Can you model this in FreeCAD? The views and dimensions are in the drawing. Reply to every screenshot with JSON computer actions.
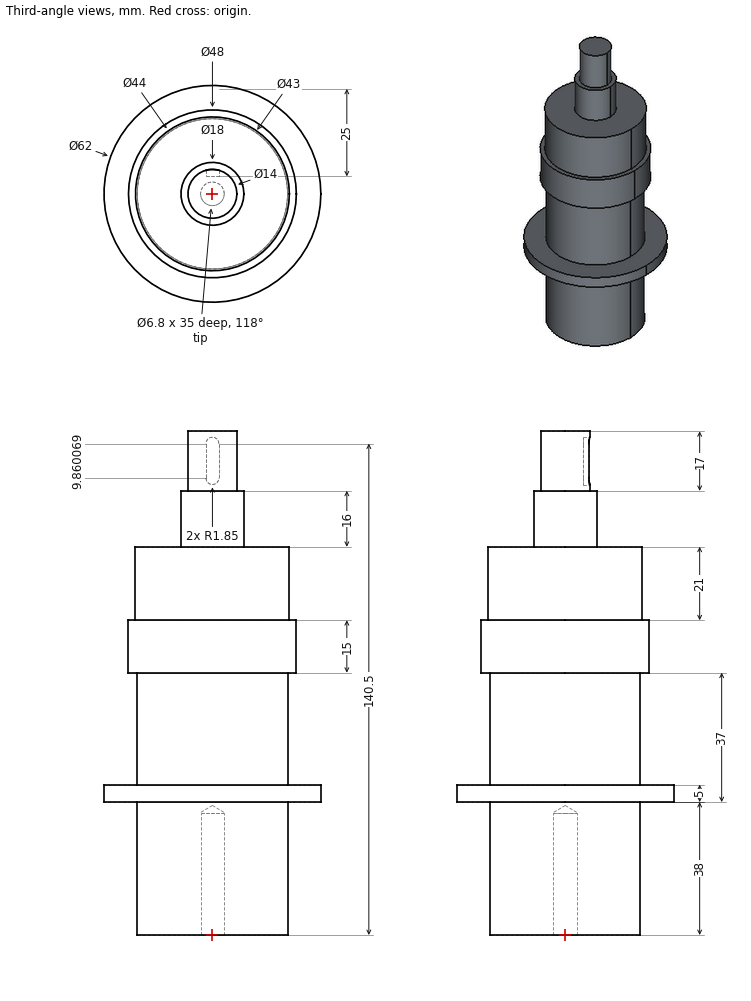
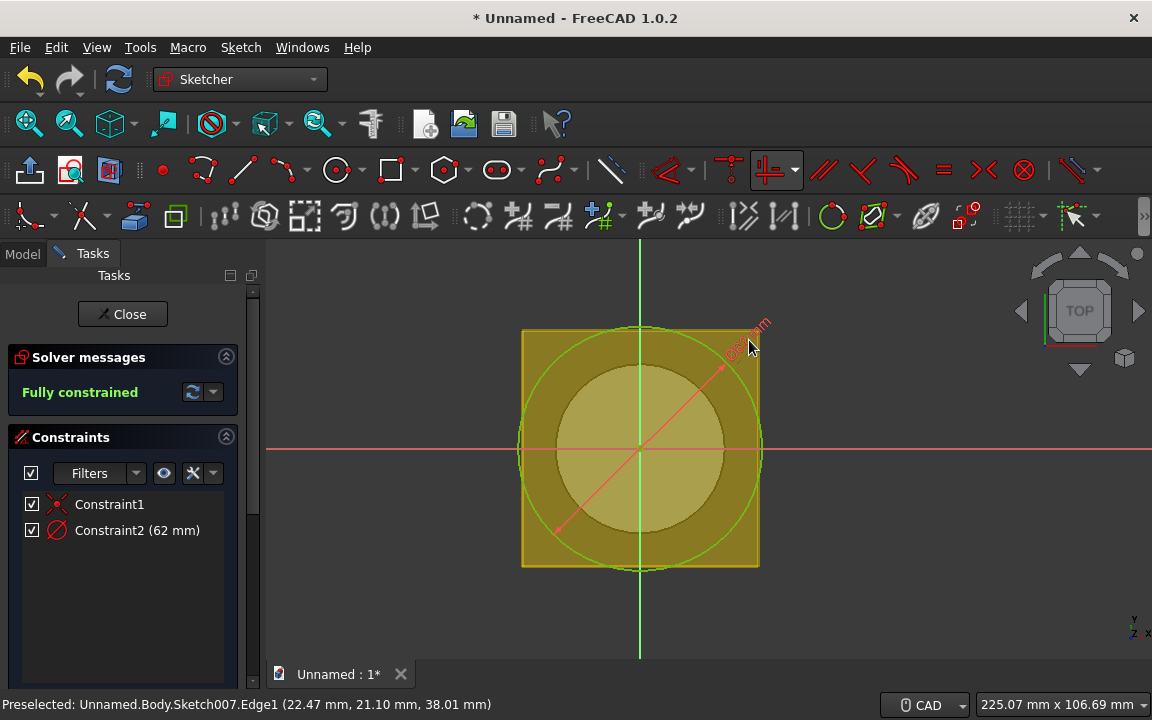
{"action": "left_click", "coordinate": [123, 314]}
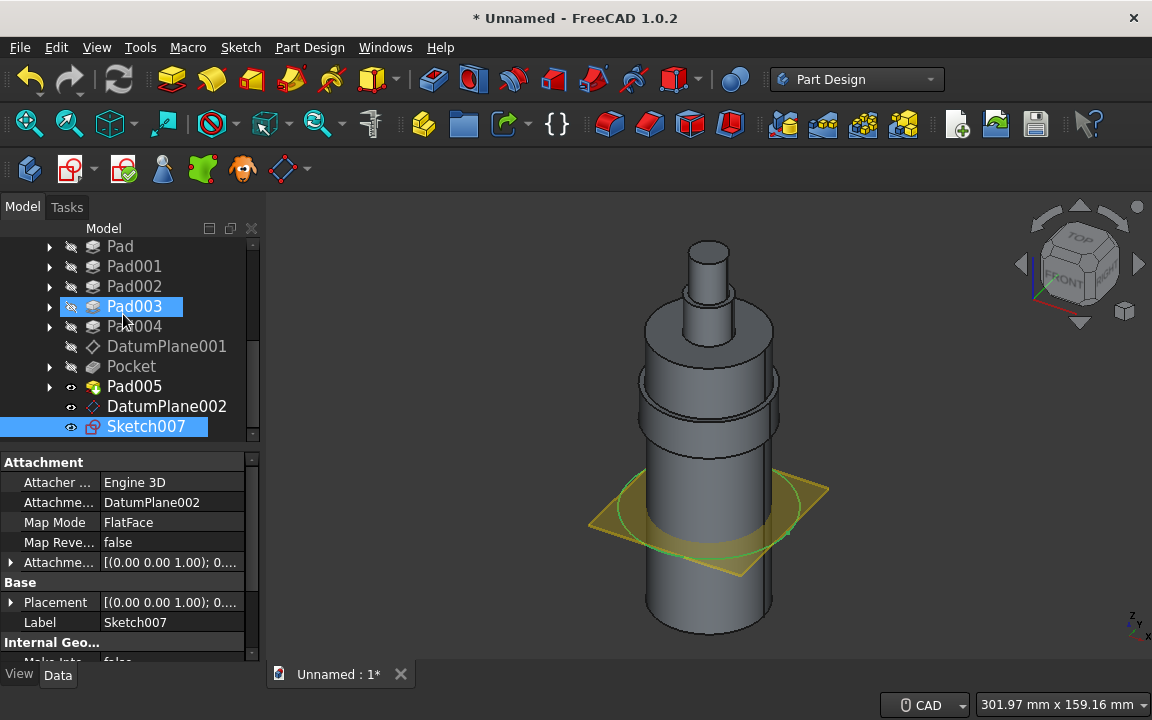
{"action": "left_click", "coordinate": [172, 80]}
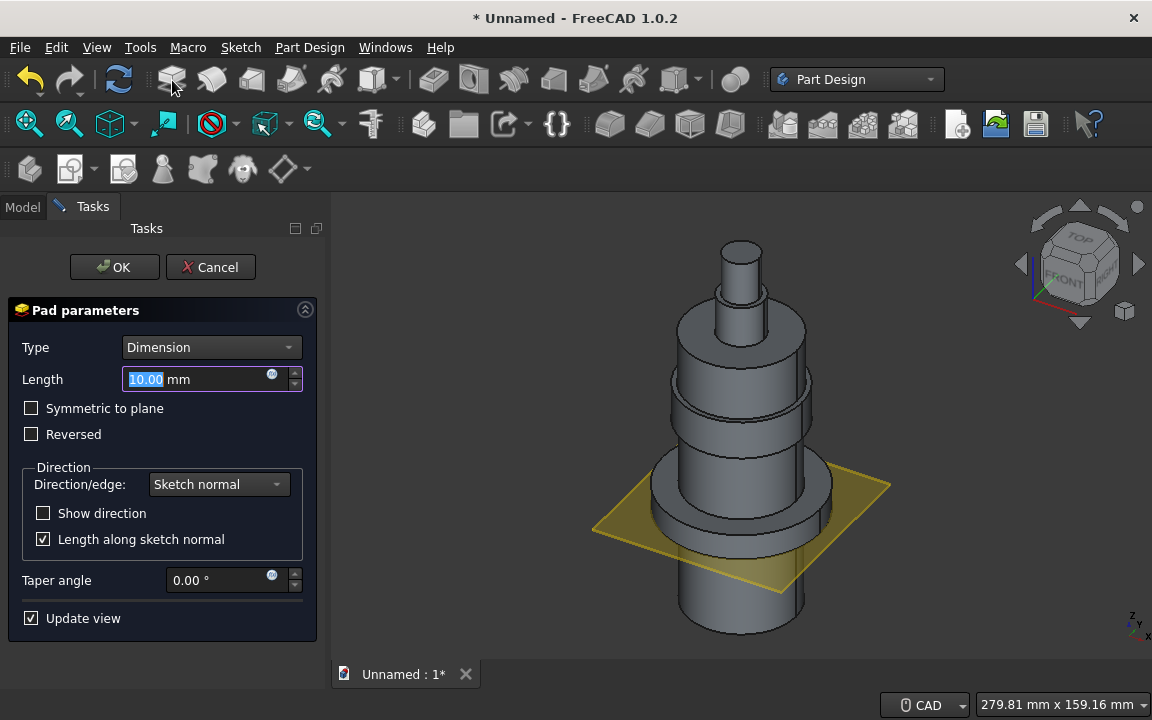
{"action": "type", "text": "5"}
{"action": "key", "text": "Tab"}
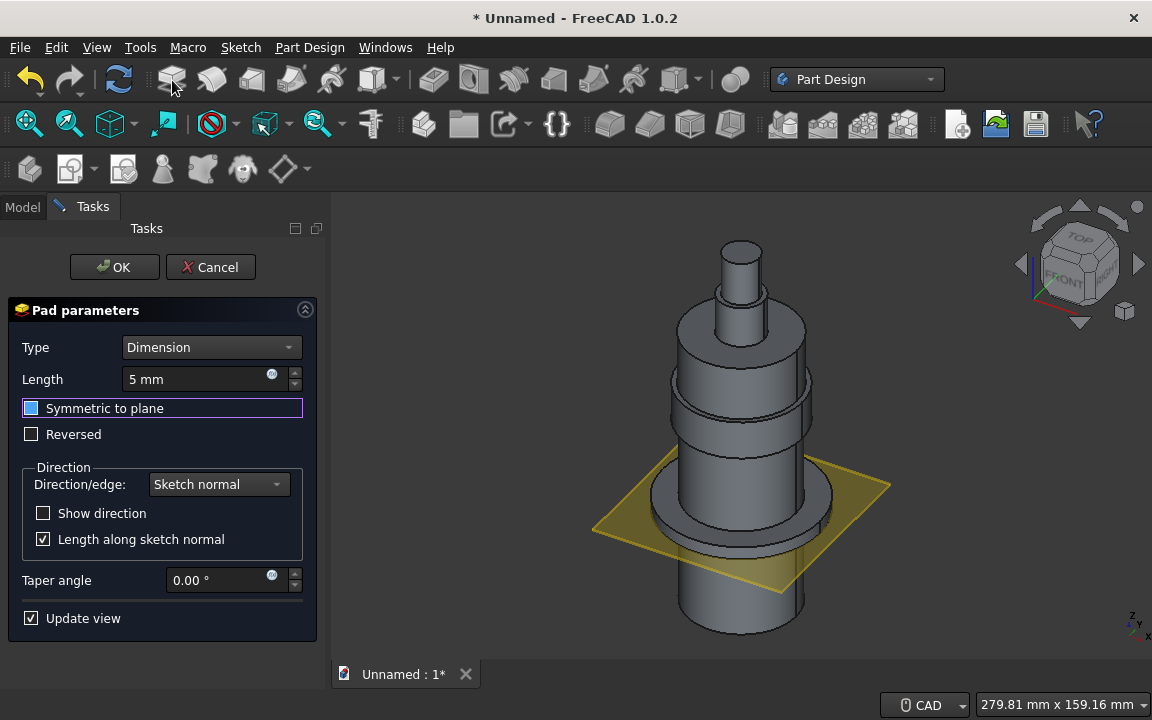
{"action": "left_click", "coordinate": [115, 267]}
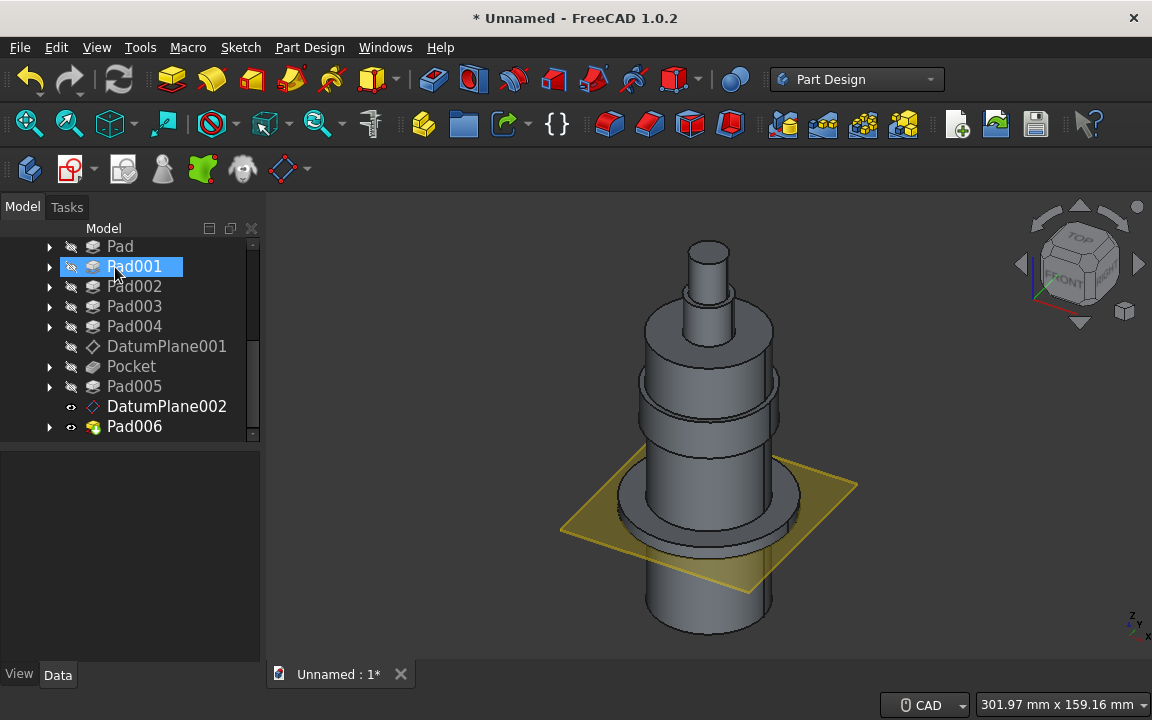
{"action": "left_click", "coordinate": [116, 407]}
{"action": "key", "text": "space"}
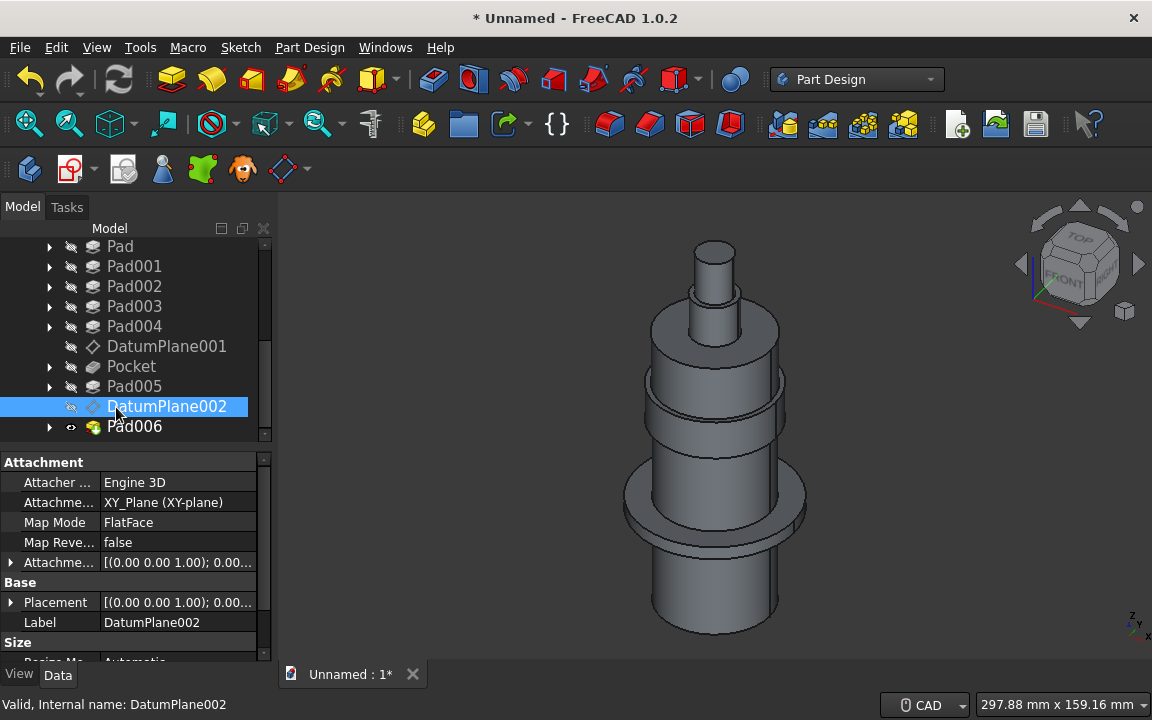
{"action": "left_click", "coordinate": [30, 124]}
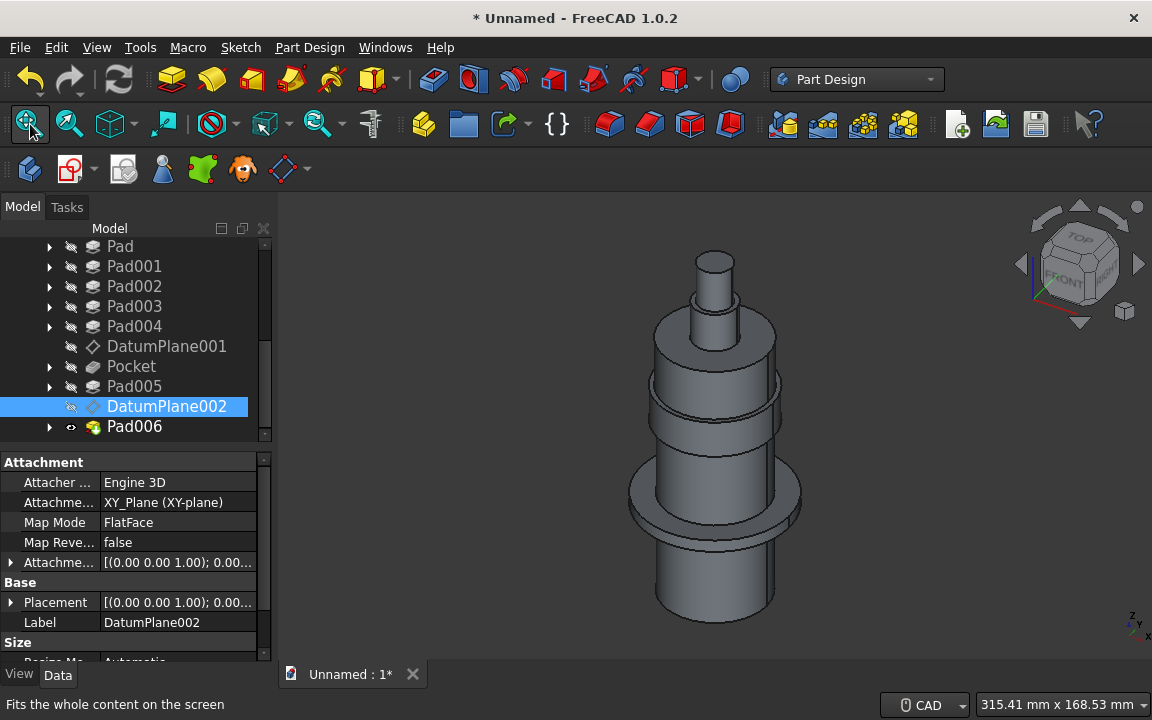
{"action": "left_click", "coordinate": [318, 619]}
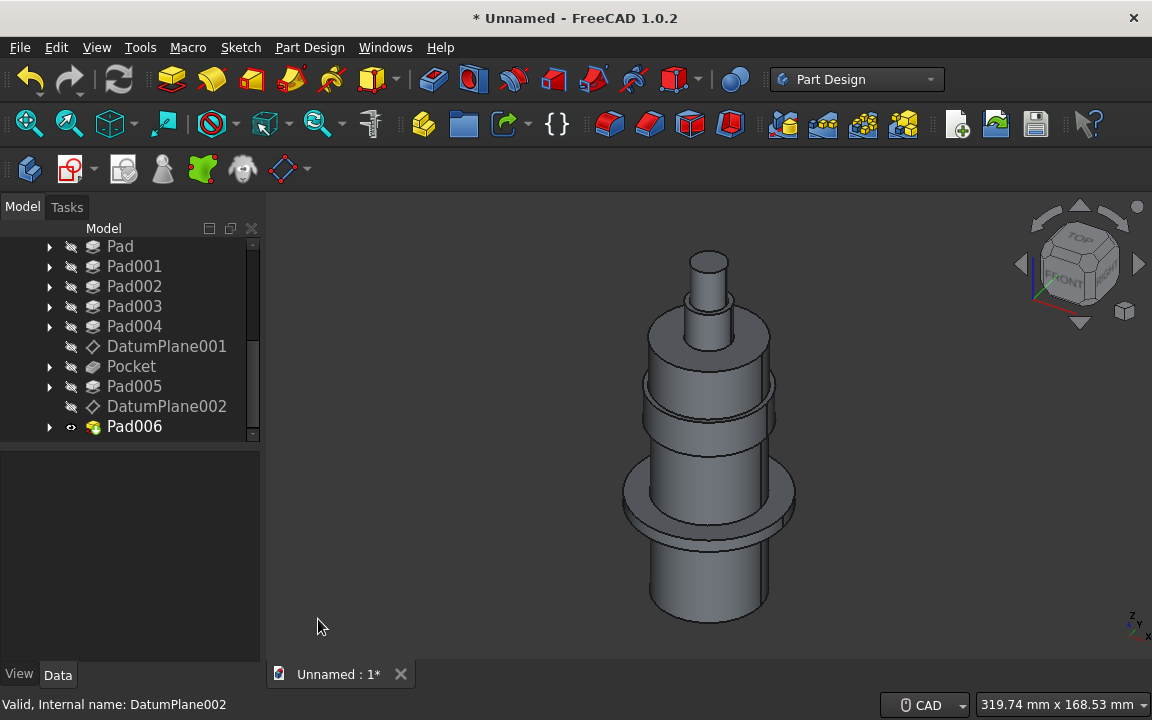
{"action": "left_click", "coordinate": [70, 170]}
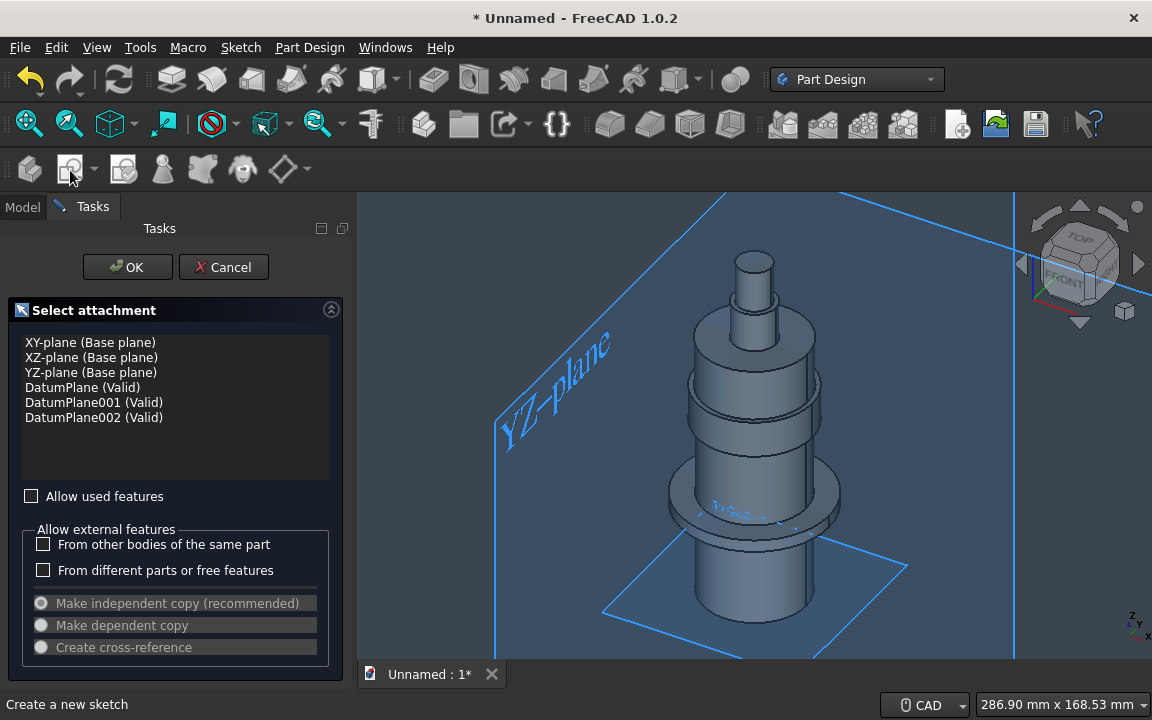
{"action": "left_click", "coordinate": [82, 342]}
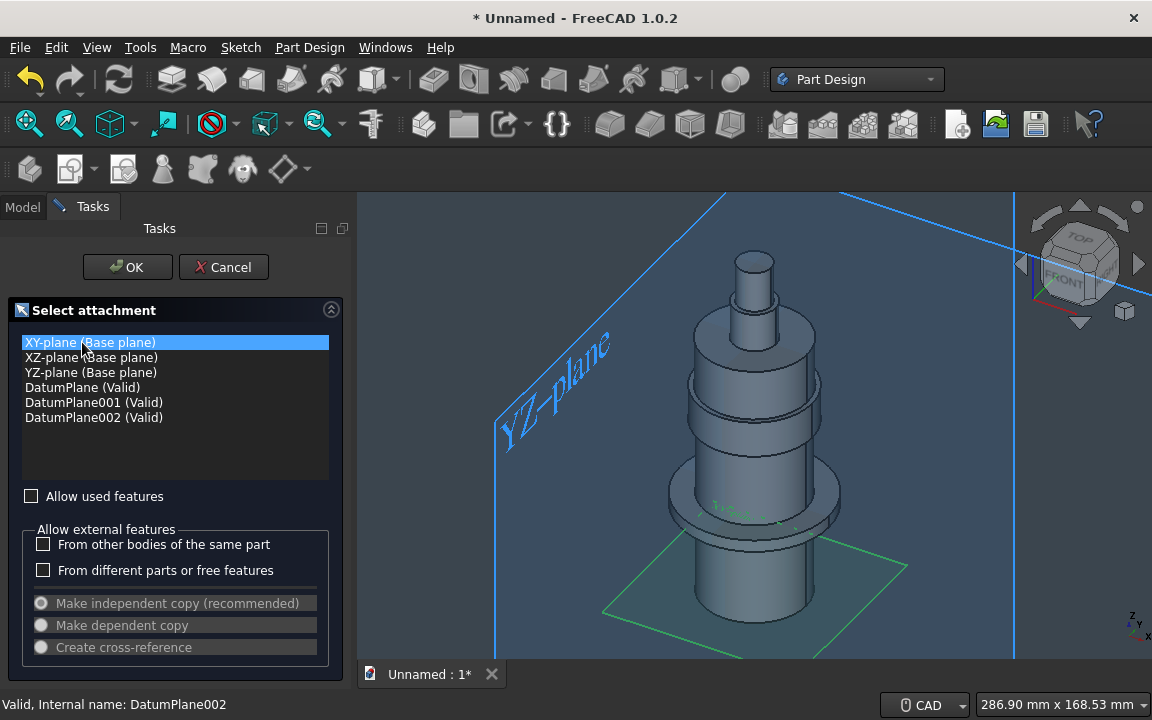
{"action": "left_click", "coordinate": [128, 267]}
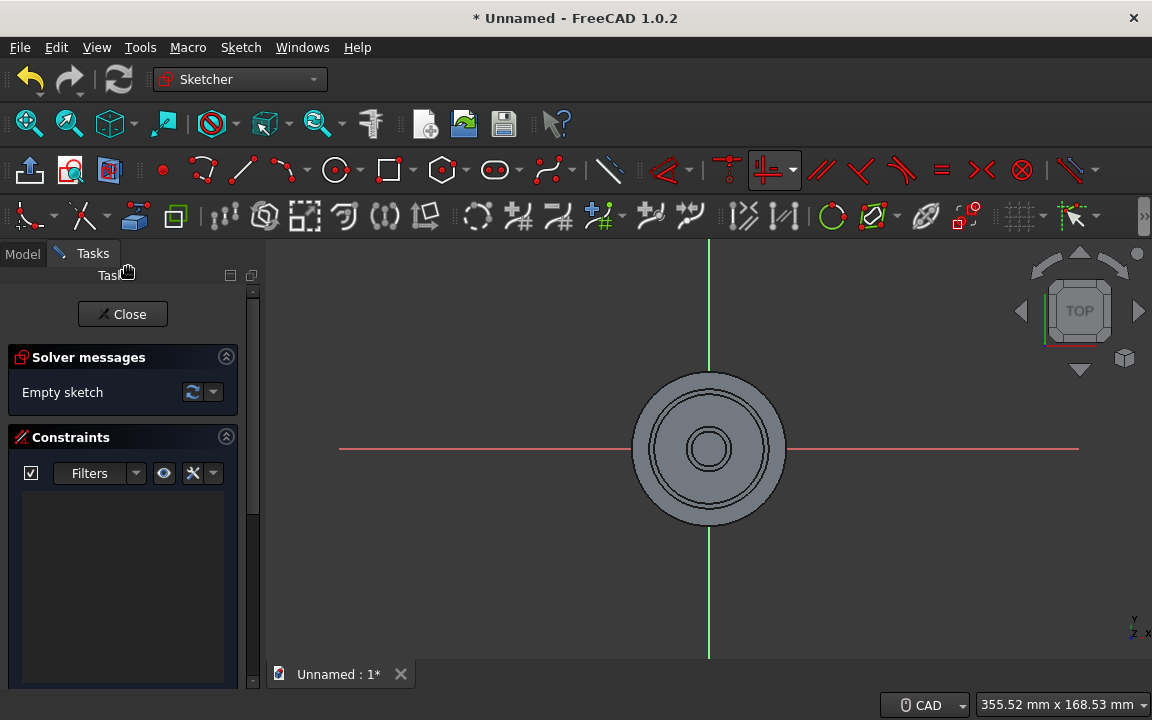
{"action": "left_click", "coordinate": [110, 170]}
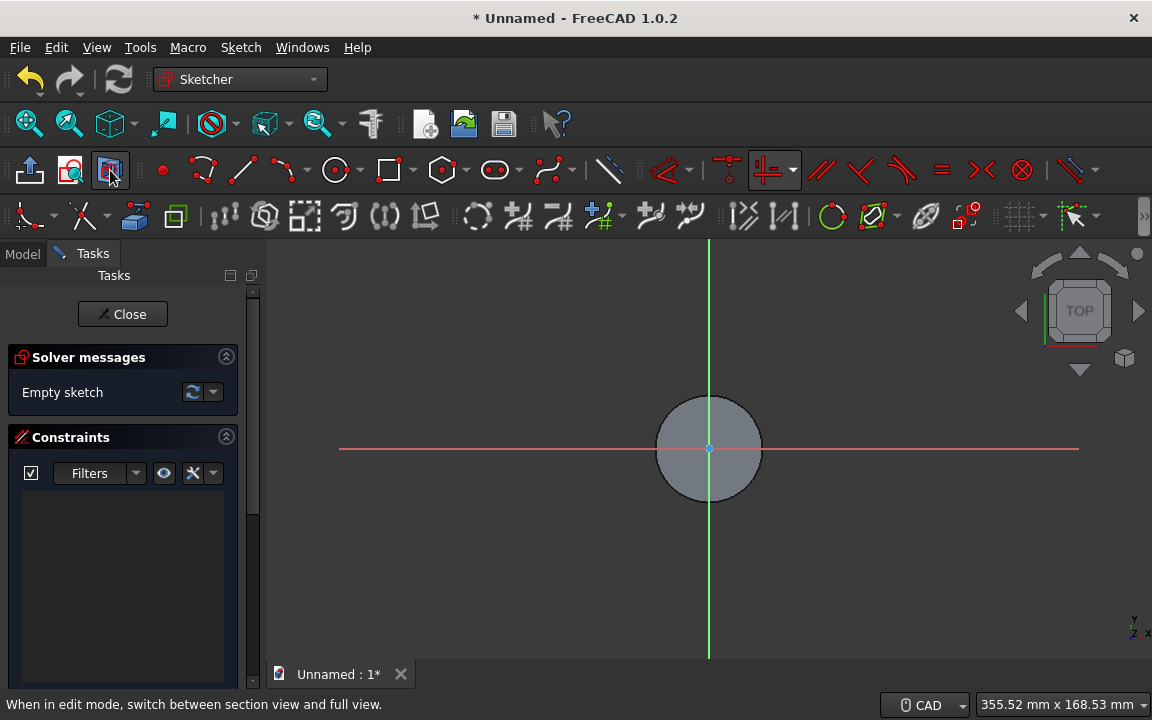
{"action": "scroll", "coordinate": [713, 449], "scroll_direction": "up", "scroll_amount": 14}